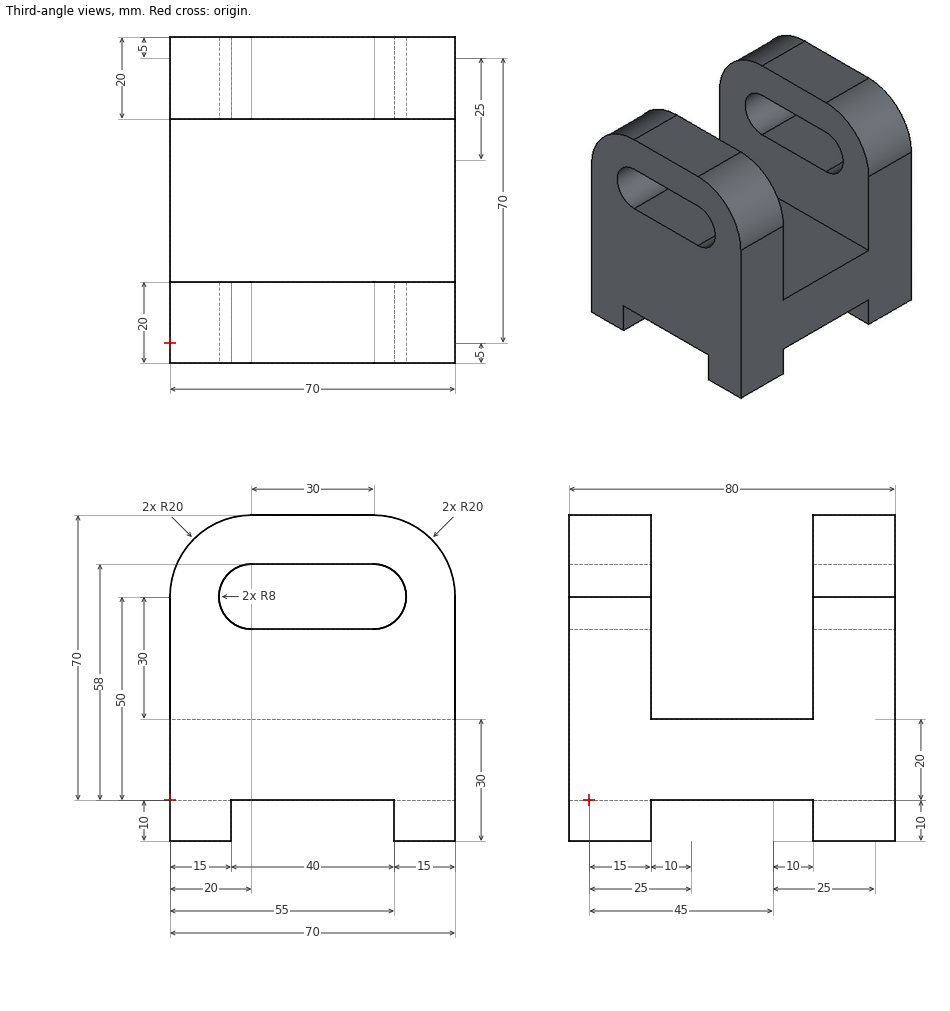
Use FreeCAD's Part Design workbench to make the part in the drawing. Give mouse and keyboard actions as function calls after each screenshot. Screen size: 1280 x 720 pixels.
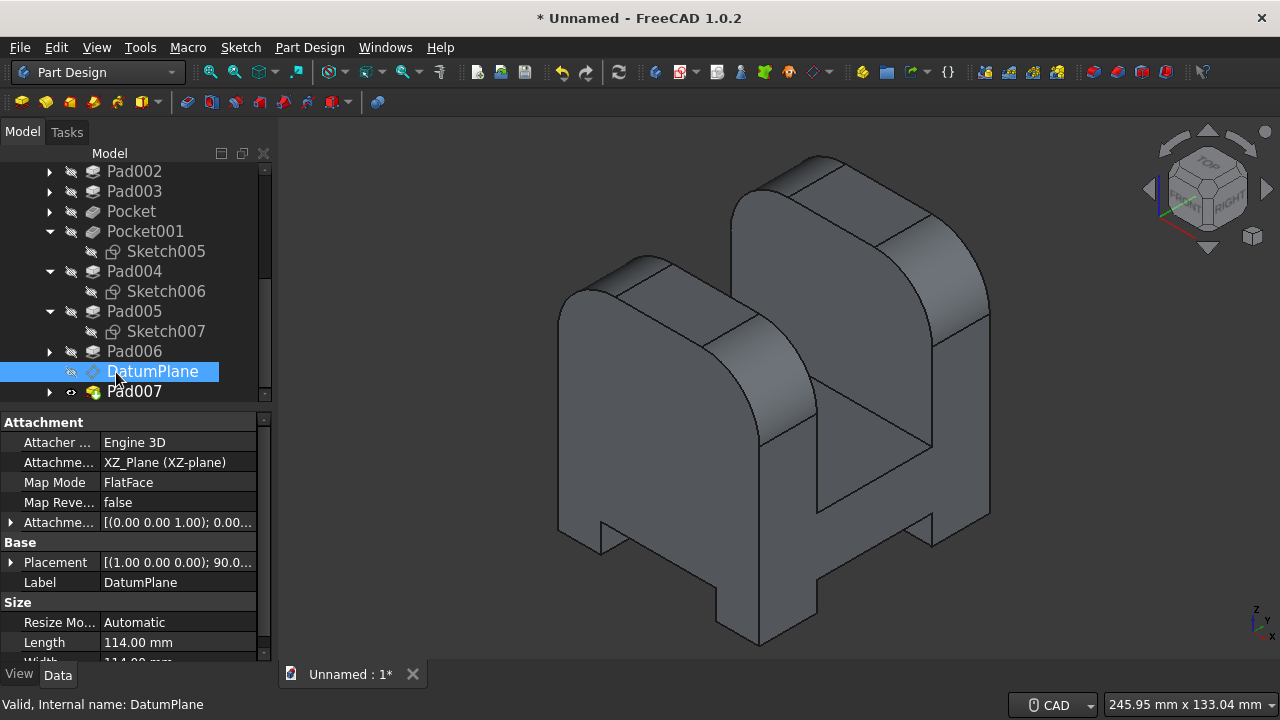
click(659, 454)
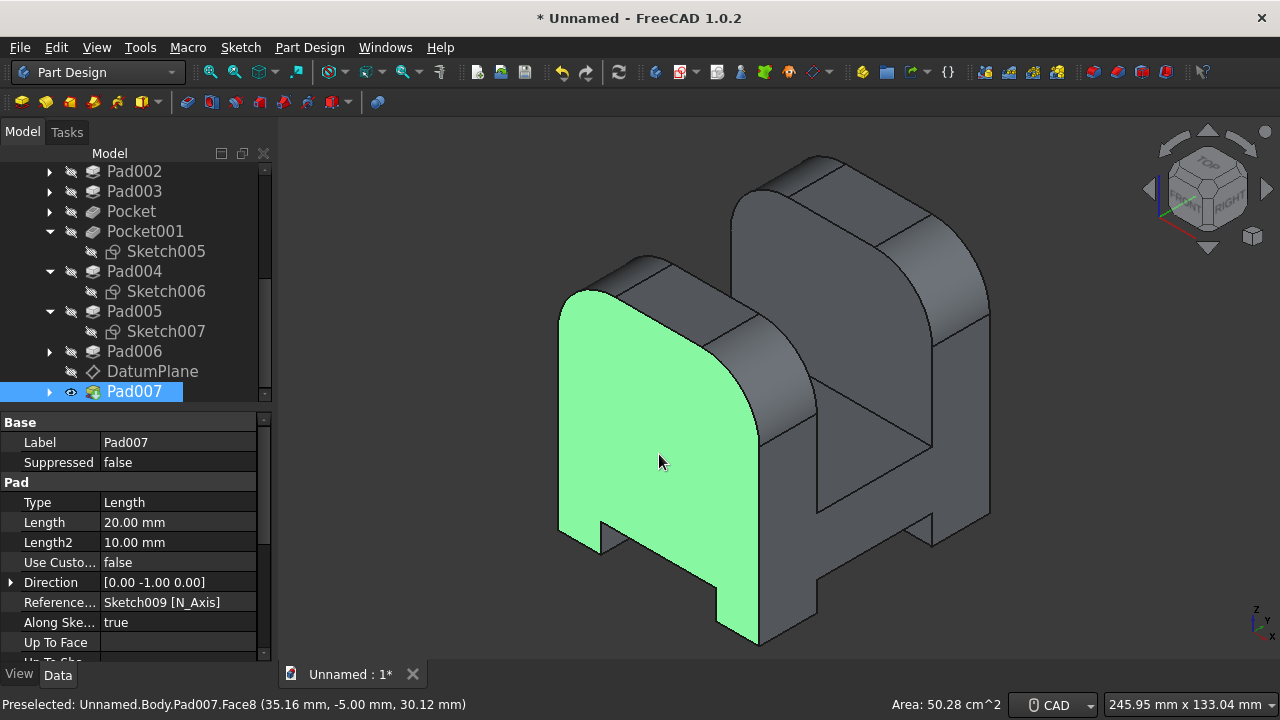
click(680, 72)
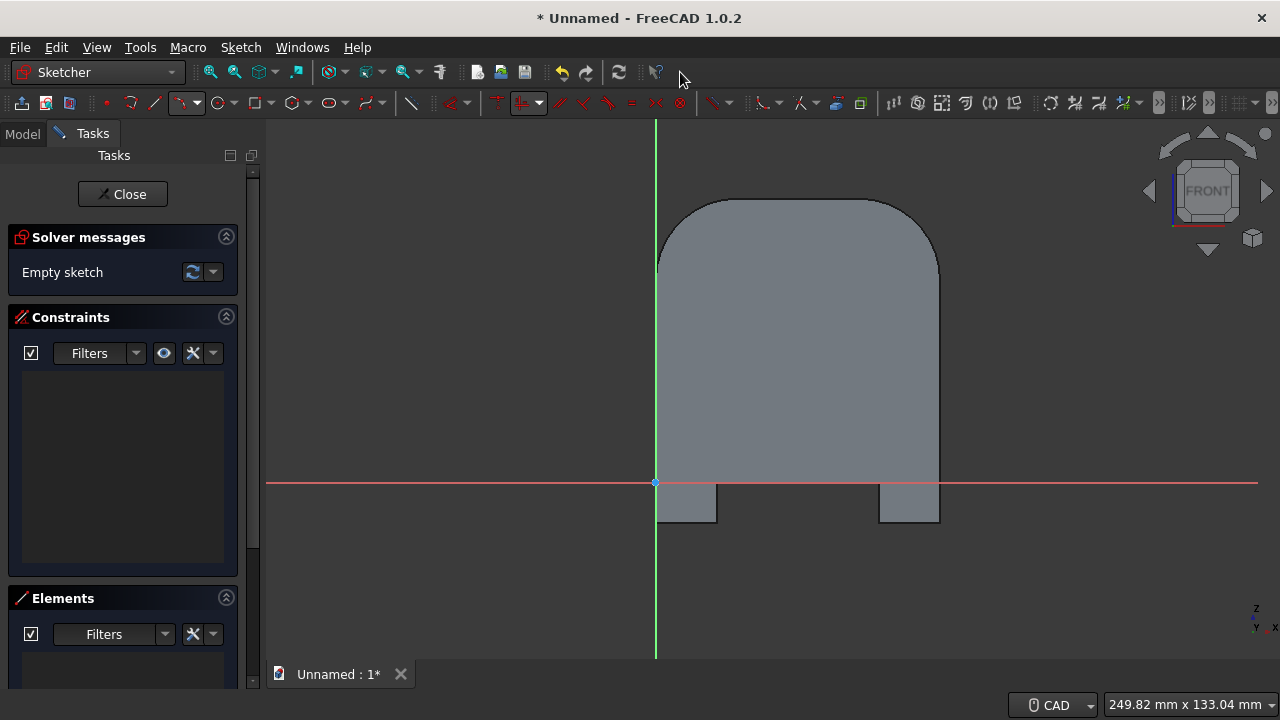
scroll(914, 317, up, 2)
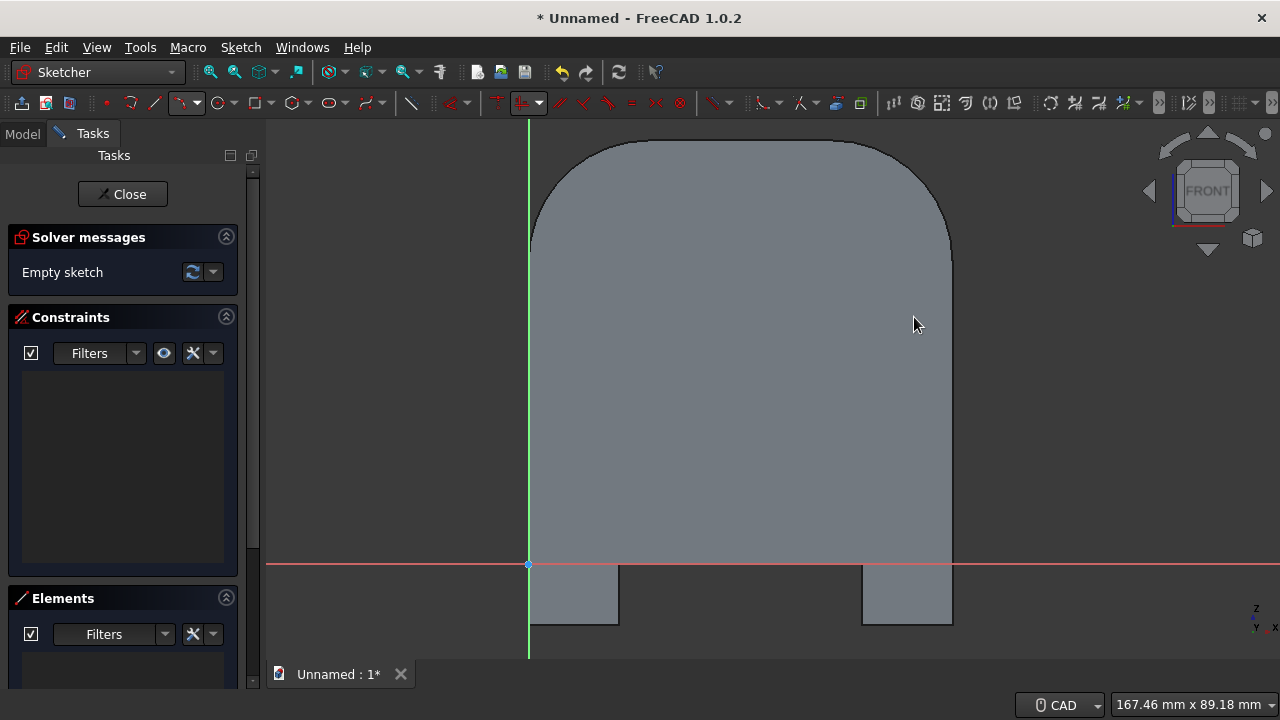
key(g)
key(s)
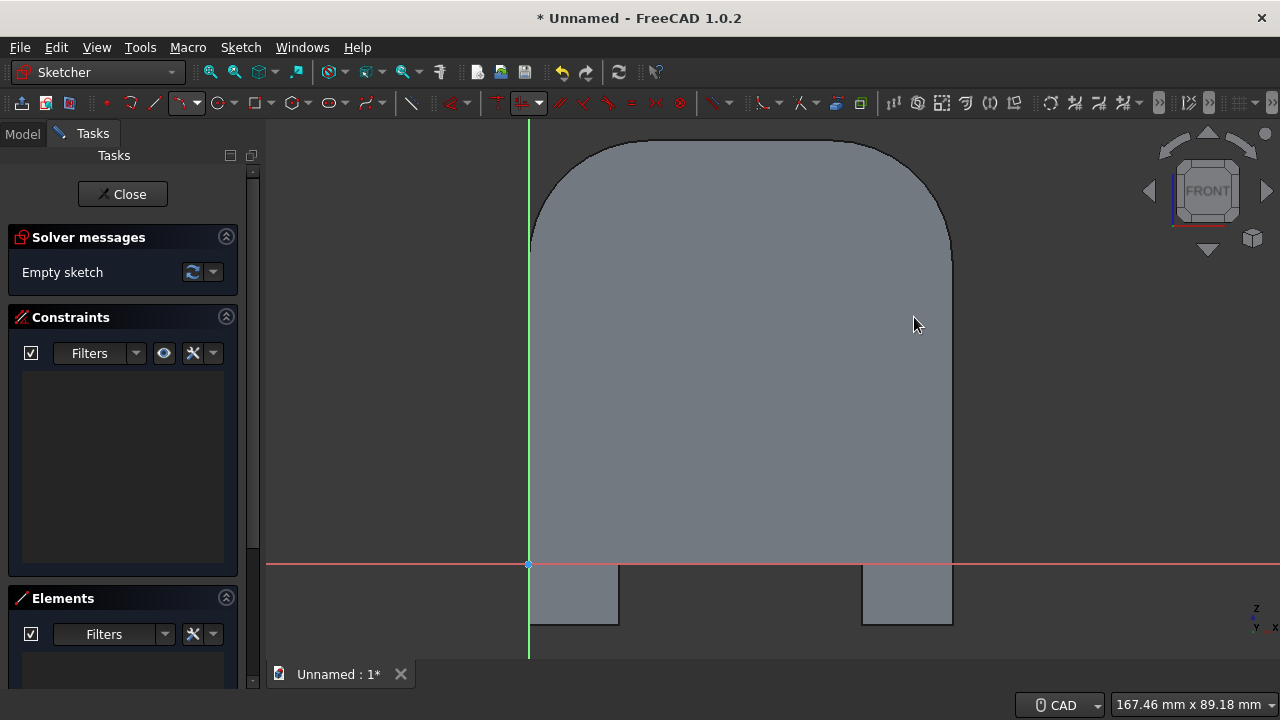
click(650, 261)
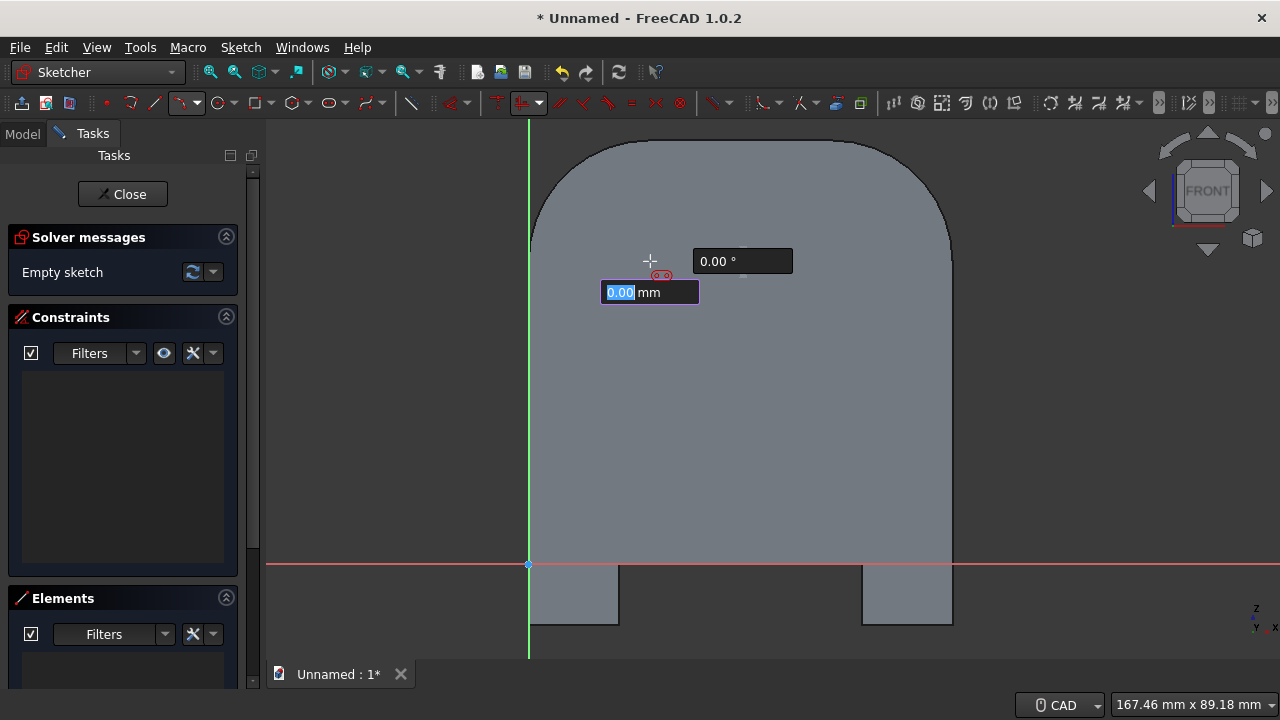
click(831, 261)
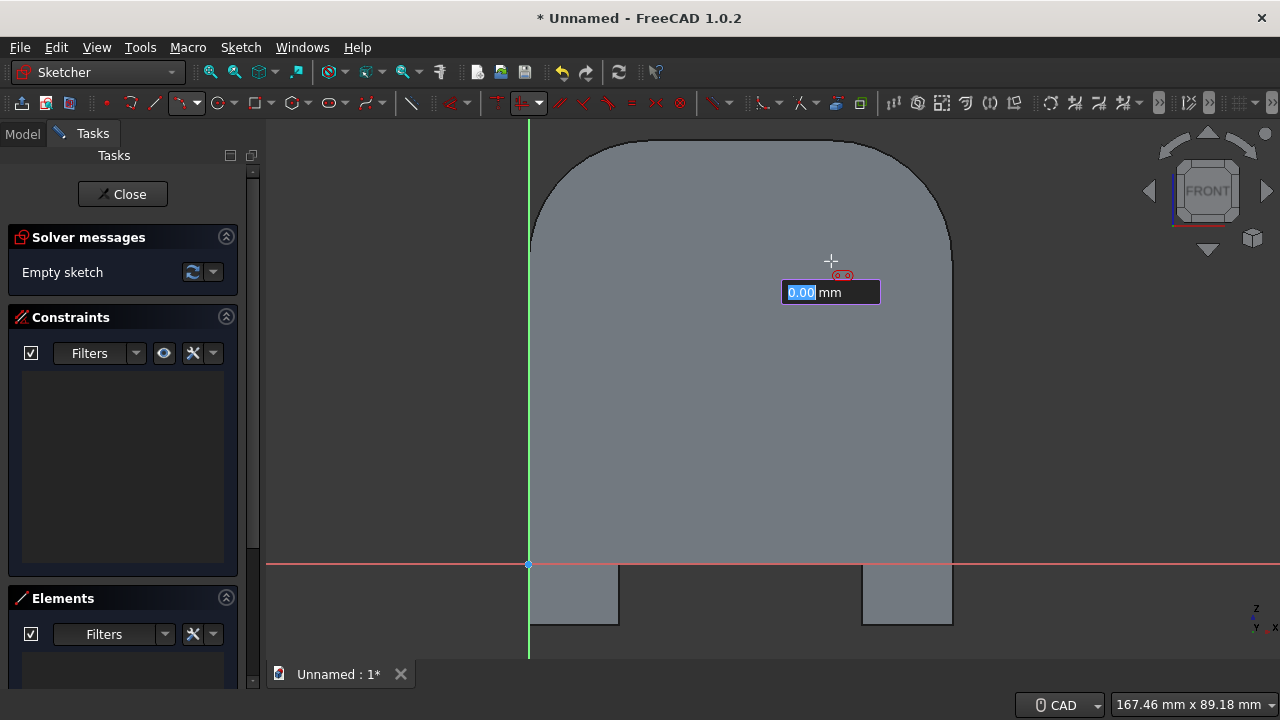
click(741, 213)
key(Escape)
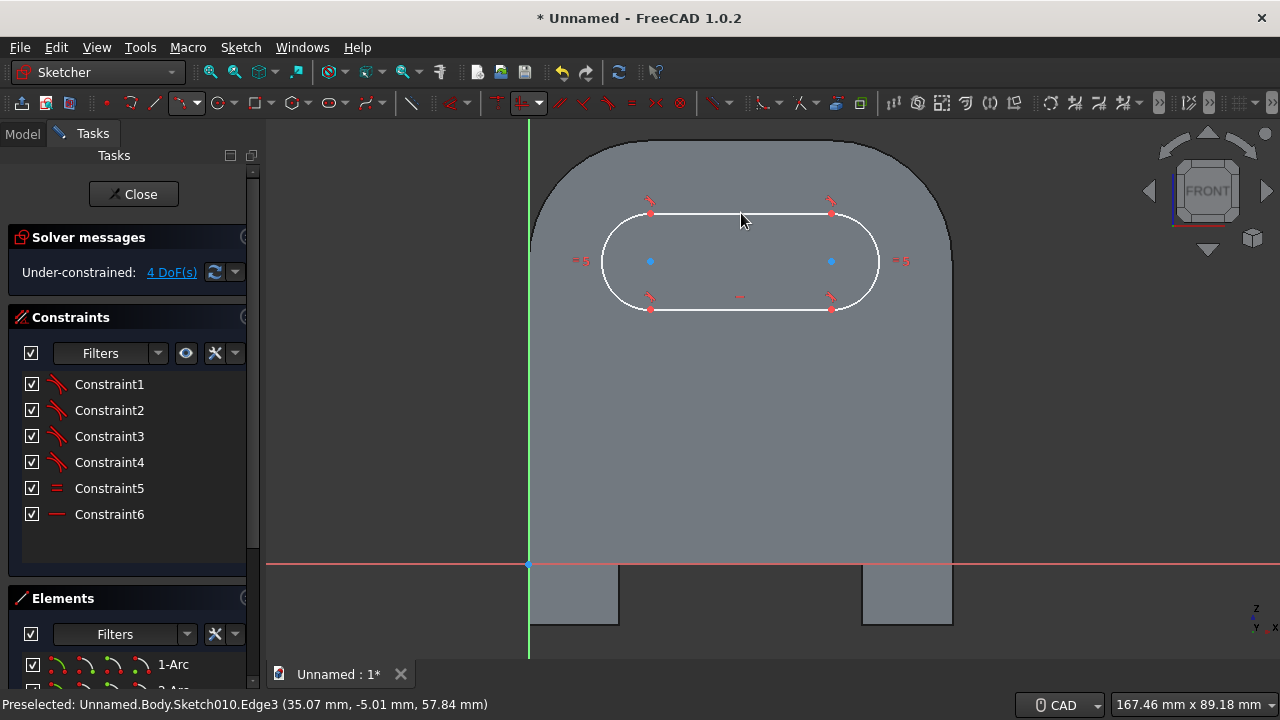
key(d)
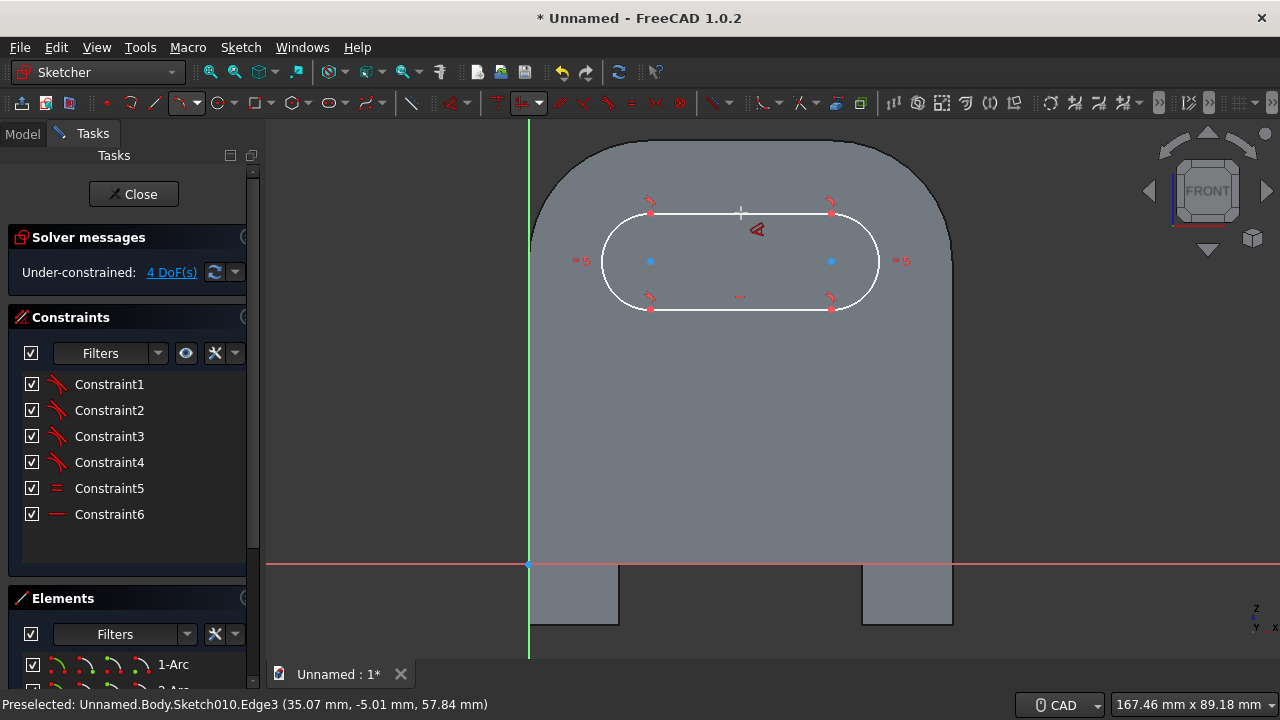
click(611, 234)
click(585, 215)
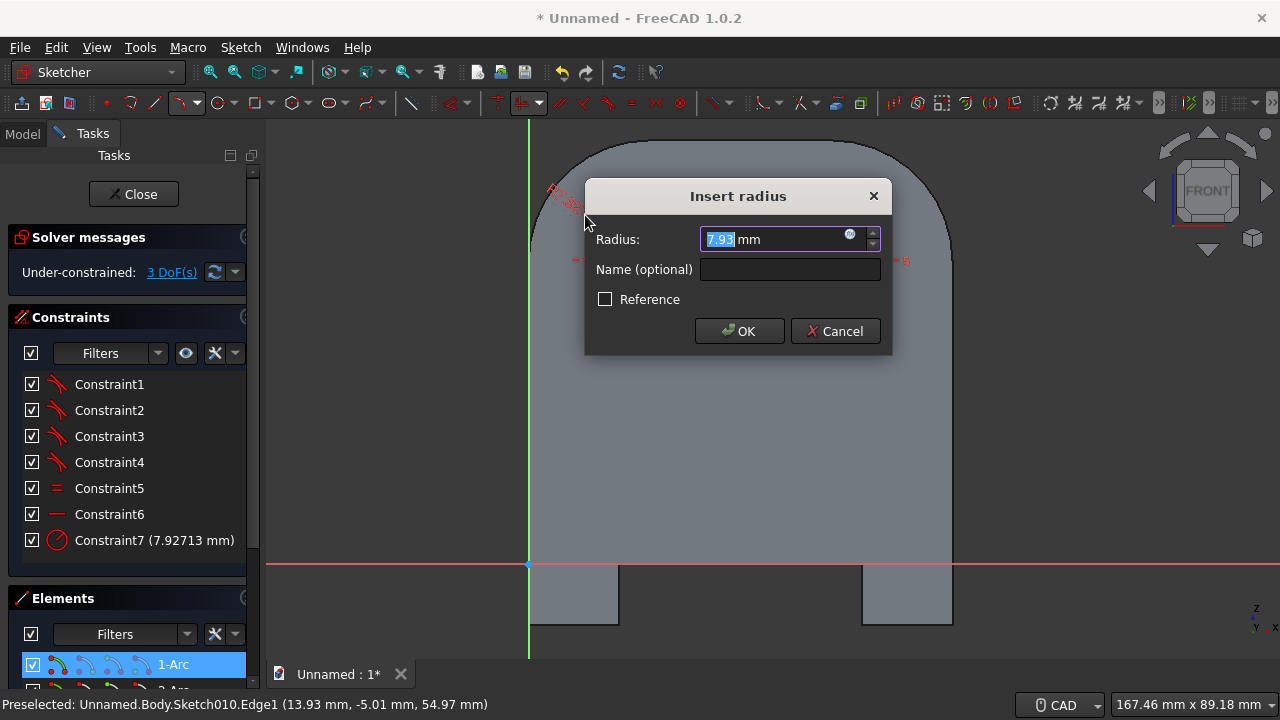
text(8)
key(Return)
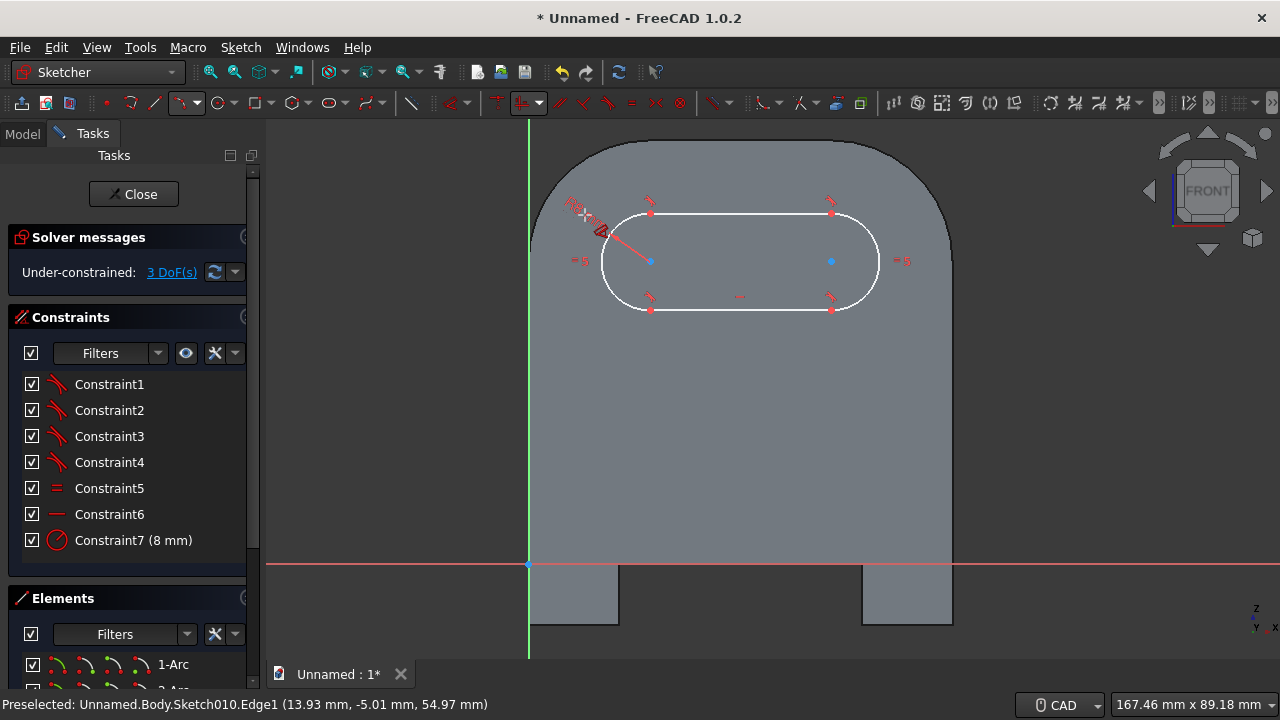
click(704, 214)
click(741, 180)